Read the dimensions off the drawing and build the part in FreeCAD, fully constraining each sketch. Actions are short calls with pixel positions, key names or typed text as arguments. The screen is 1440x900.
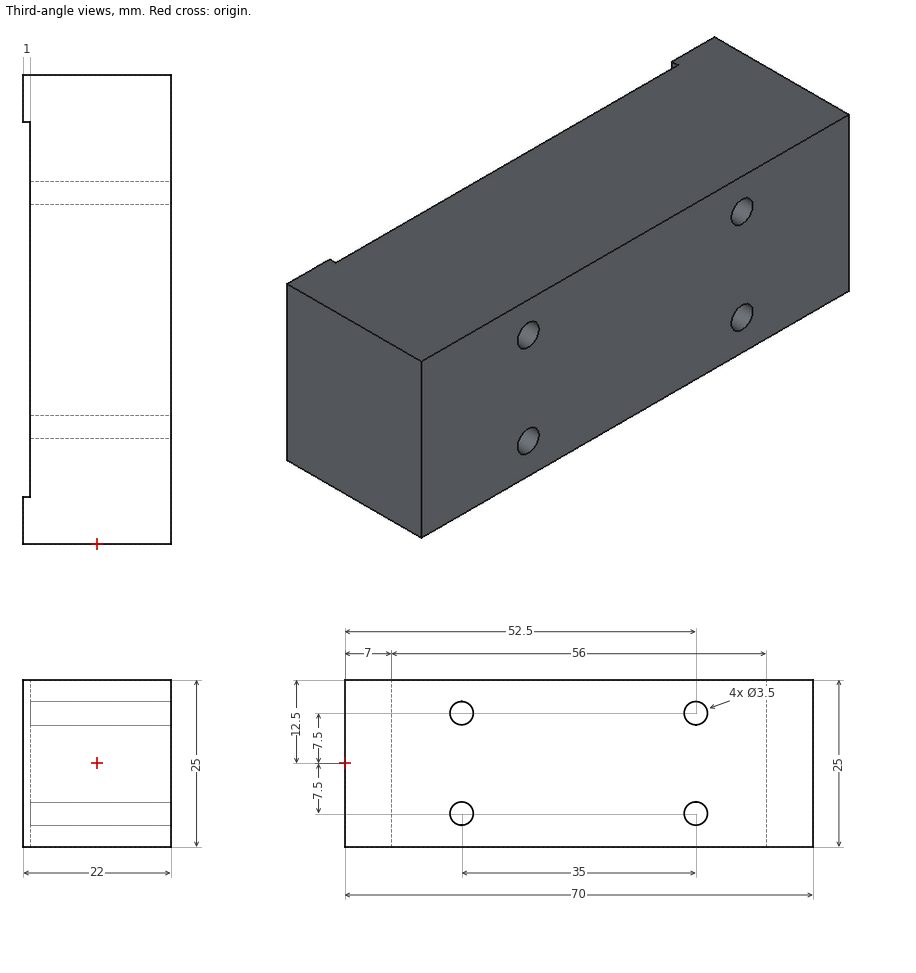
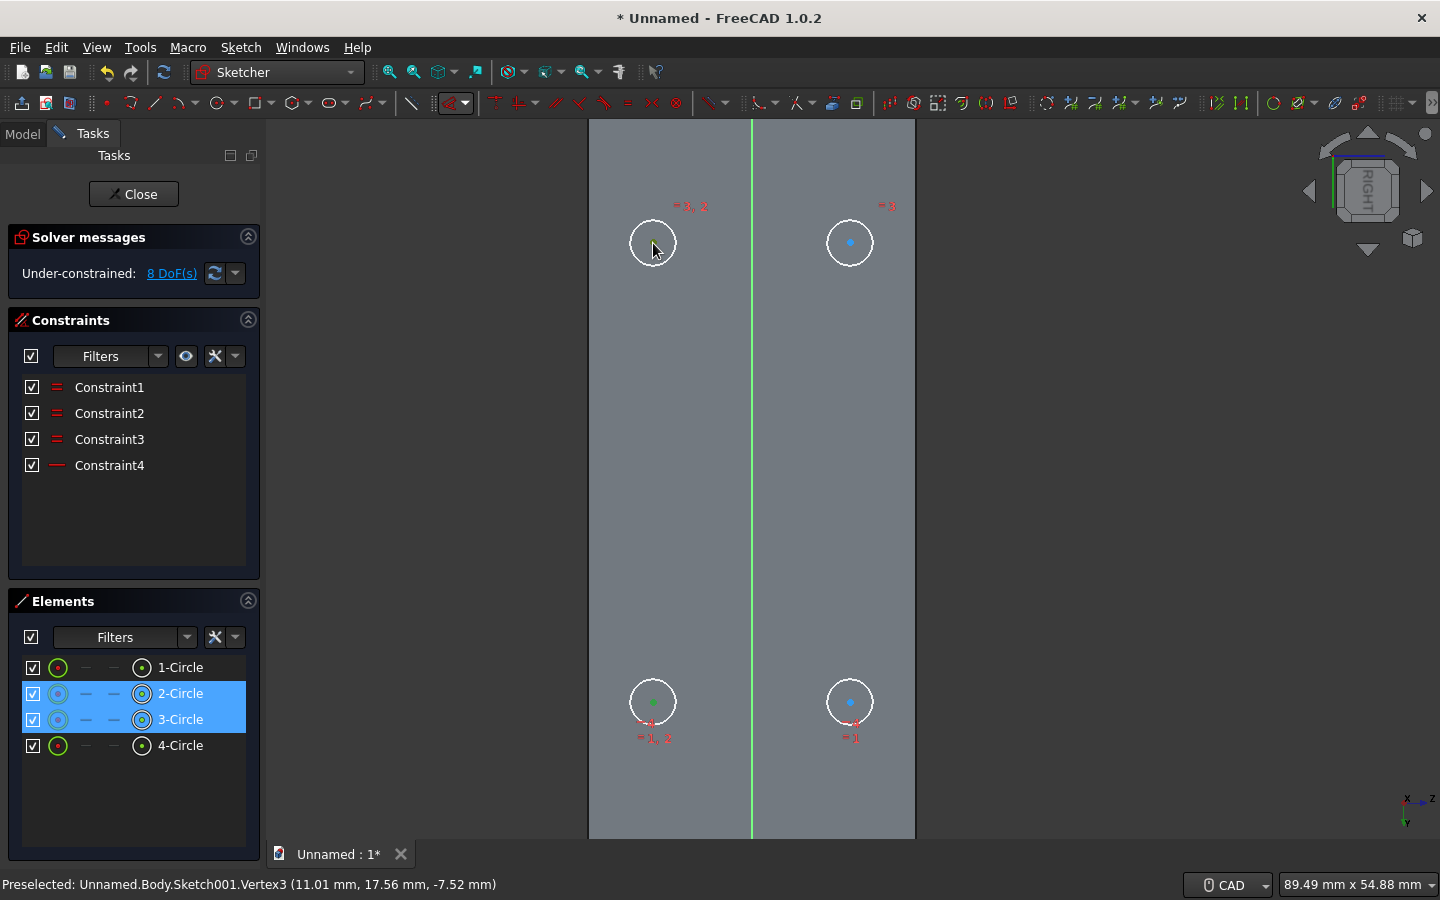
click(538, 104)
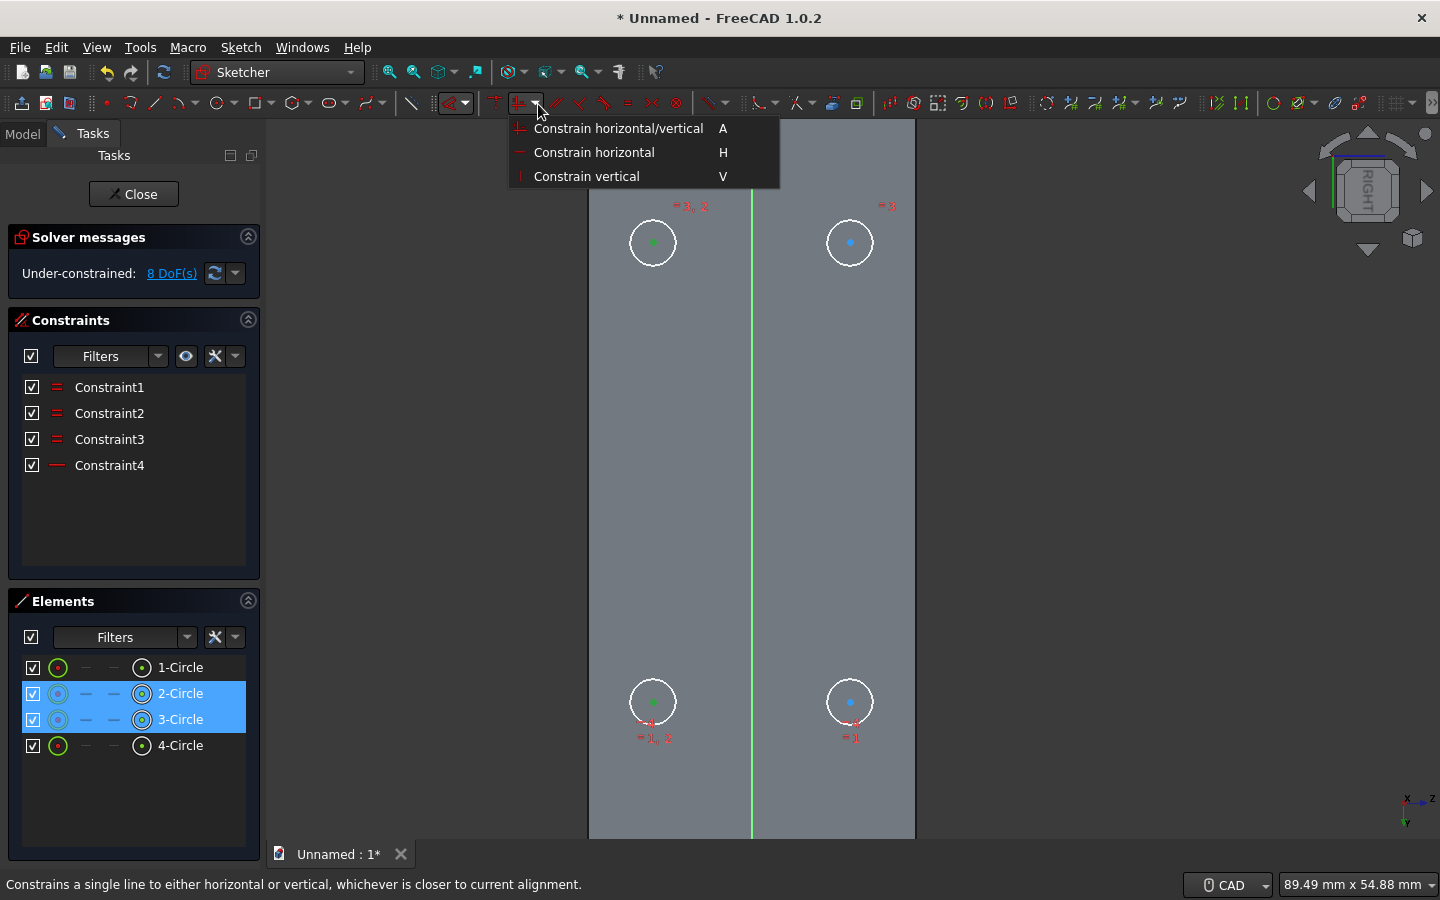
click(644, 176)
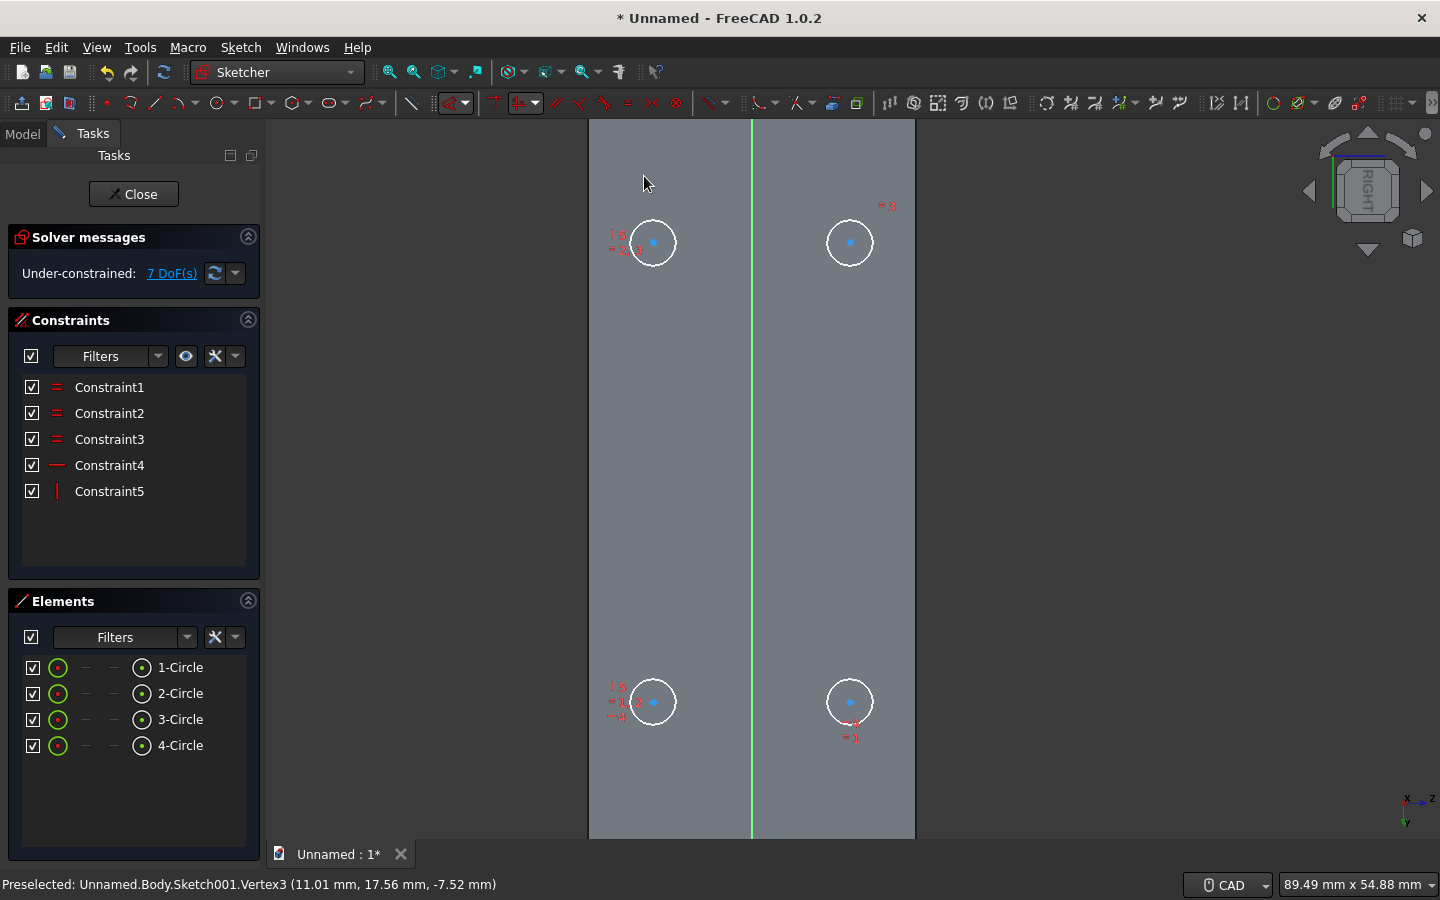
click(850, 702)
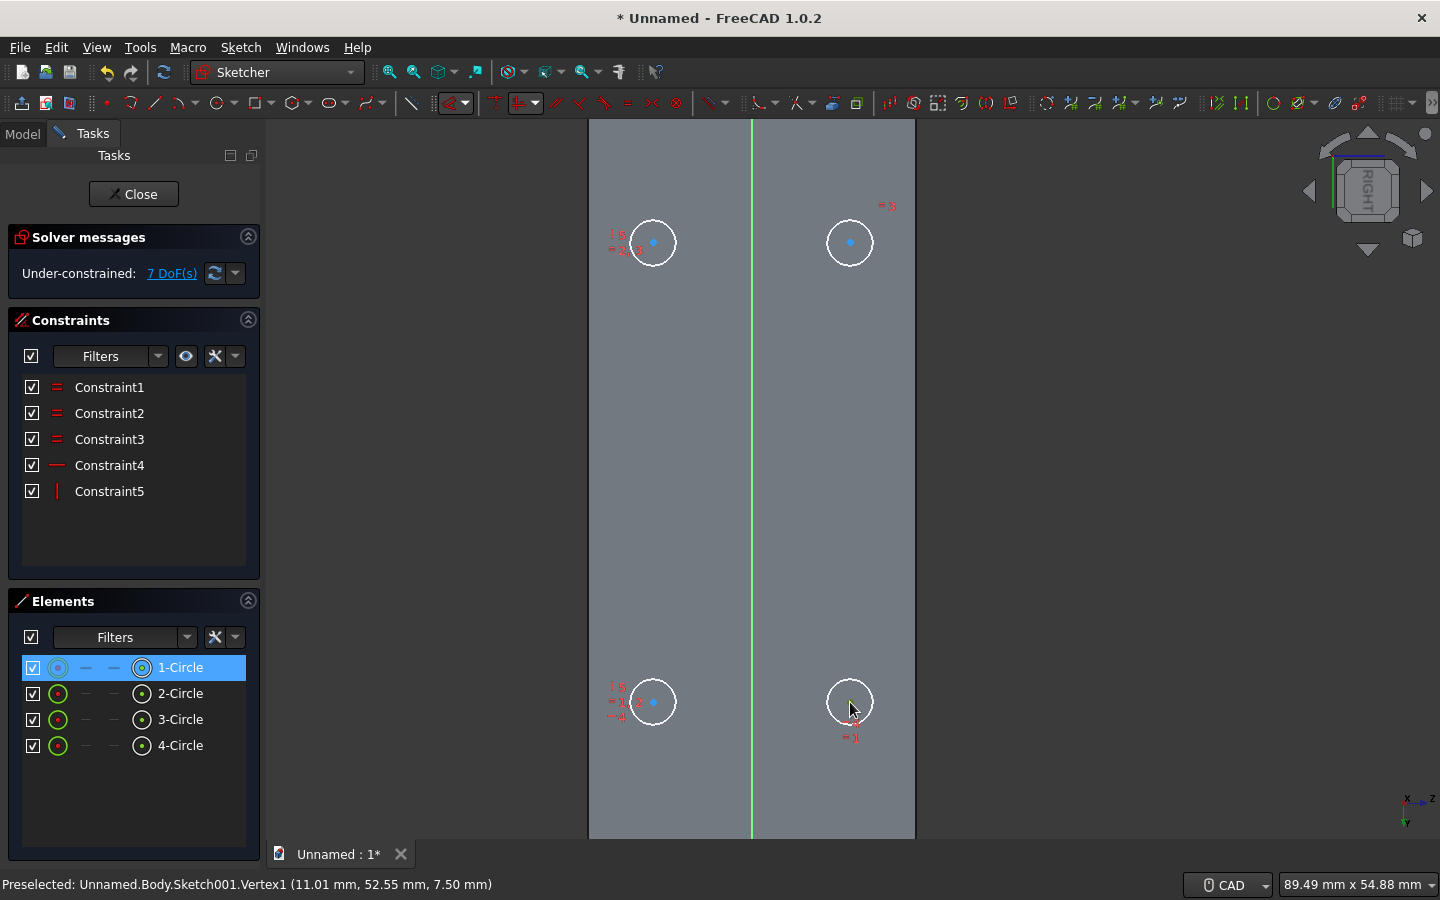
click(850, 243)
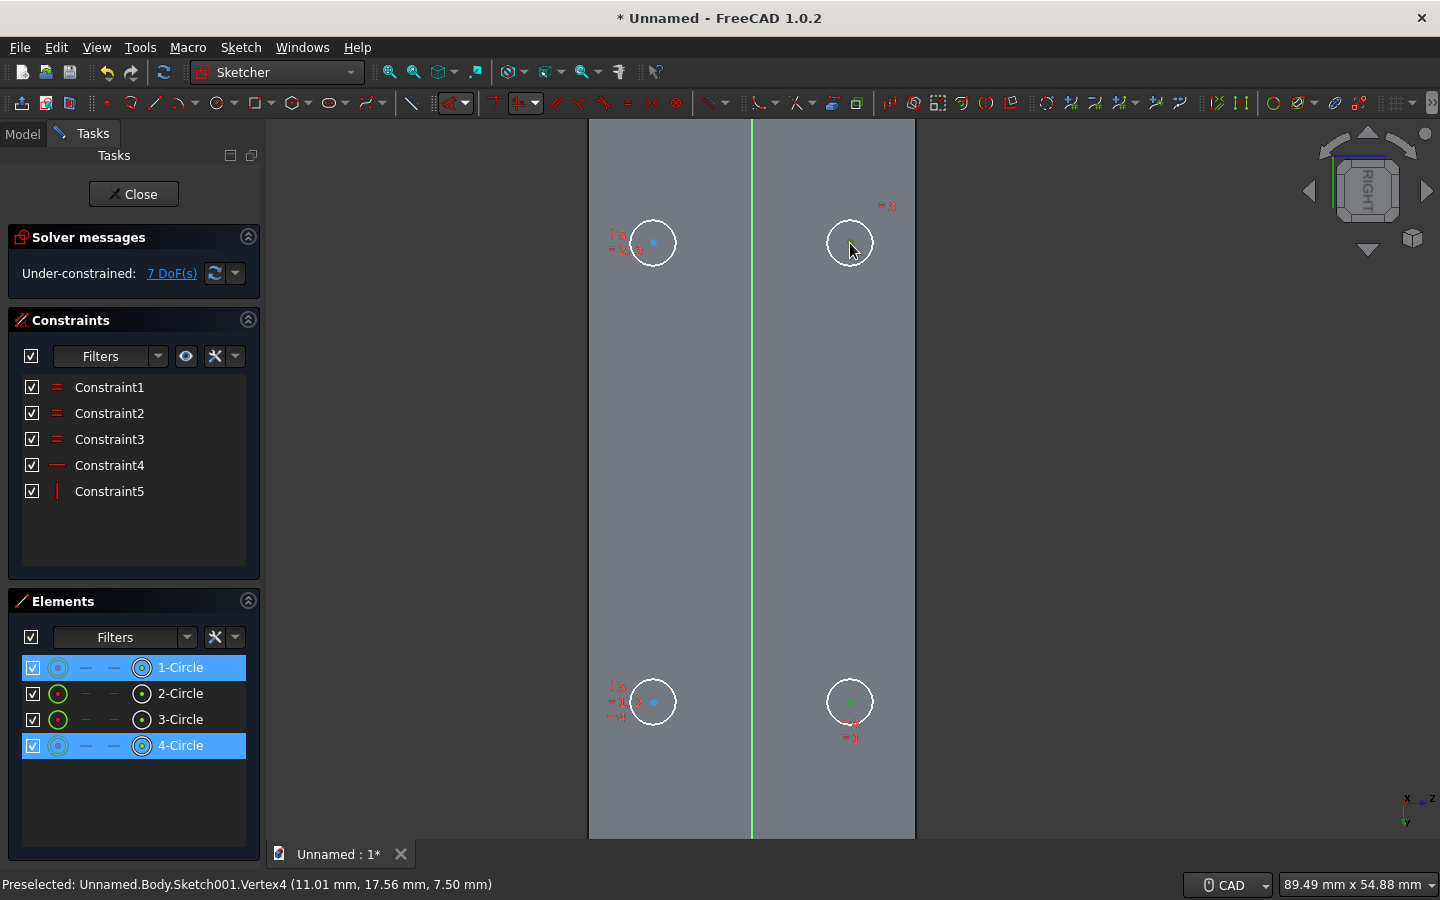
key(v)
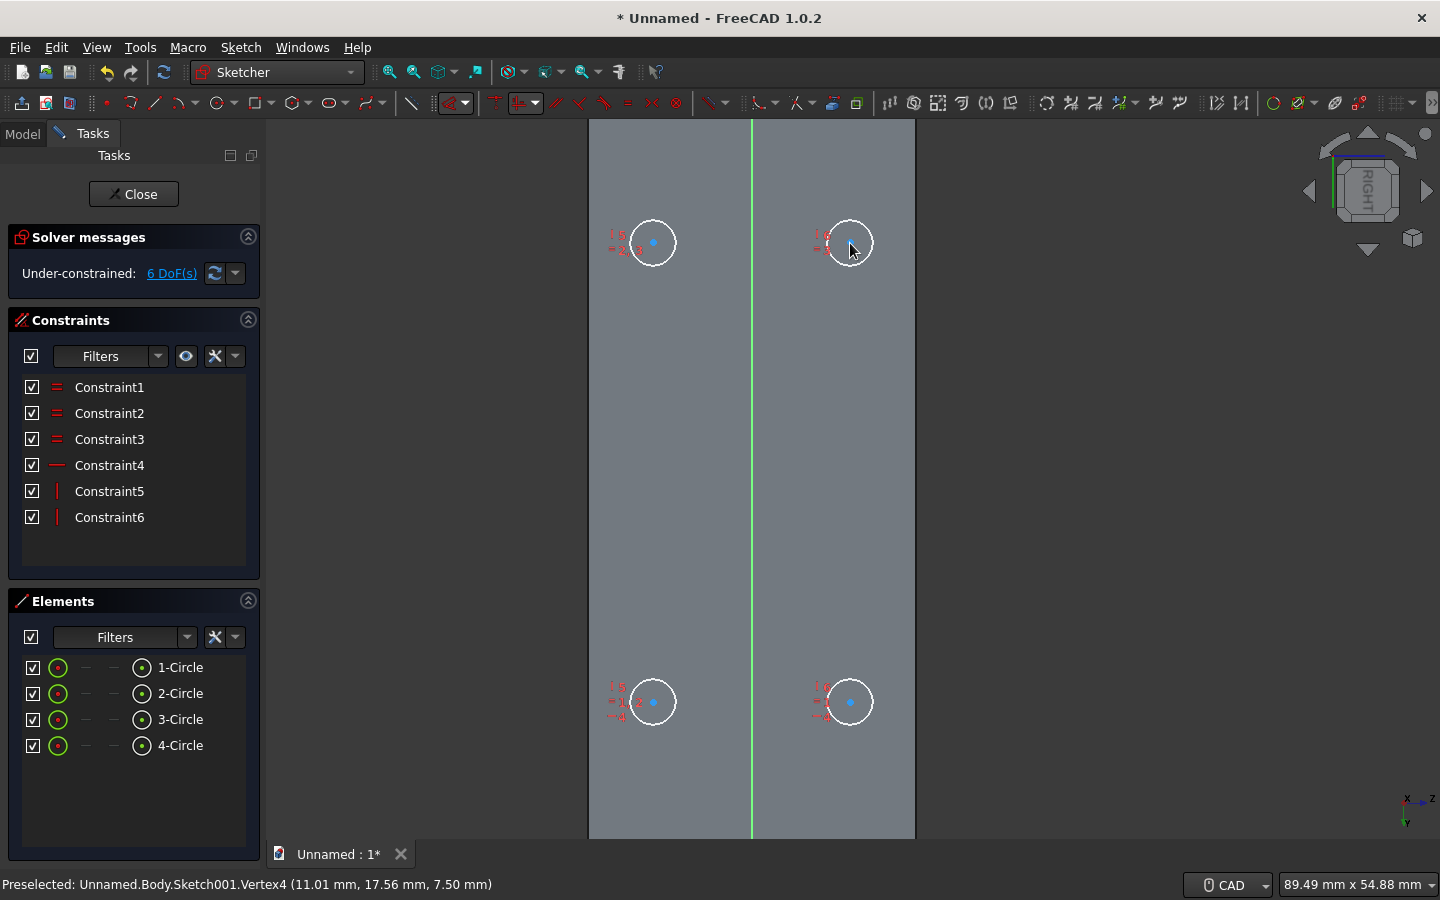
click(653, 243)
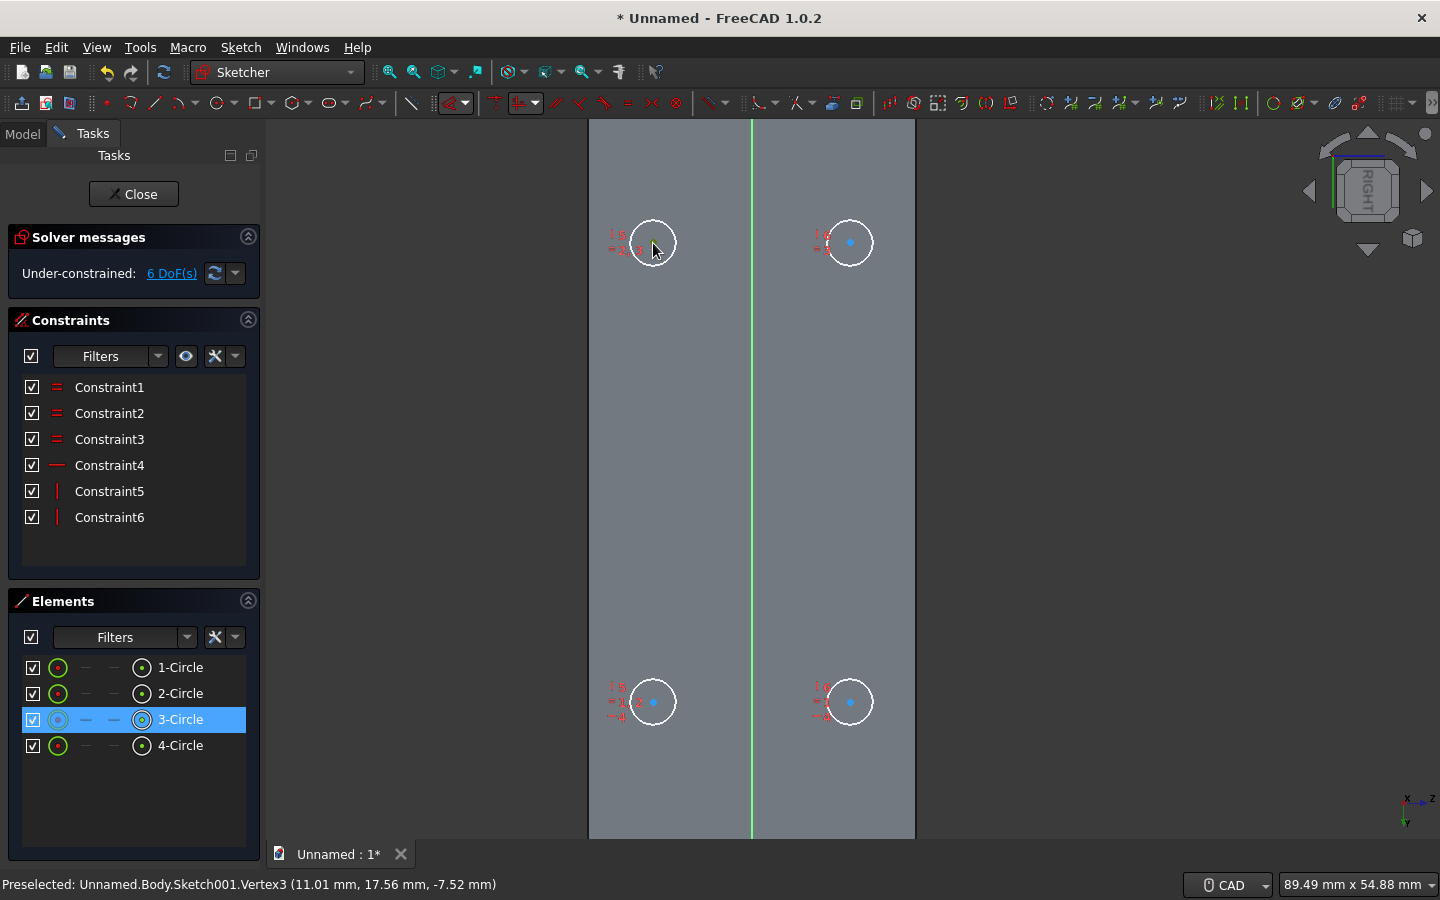
click(850, 243)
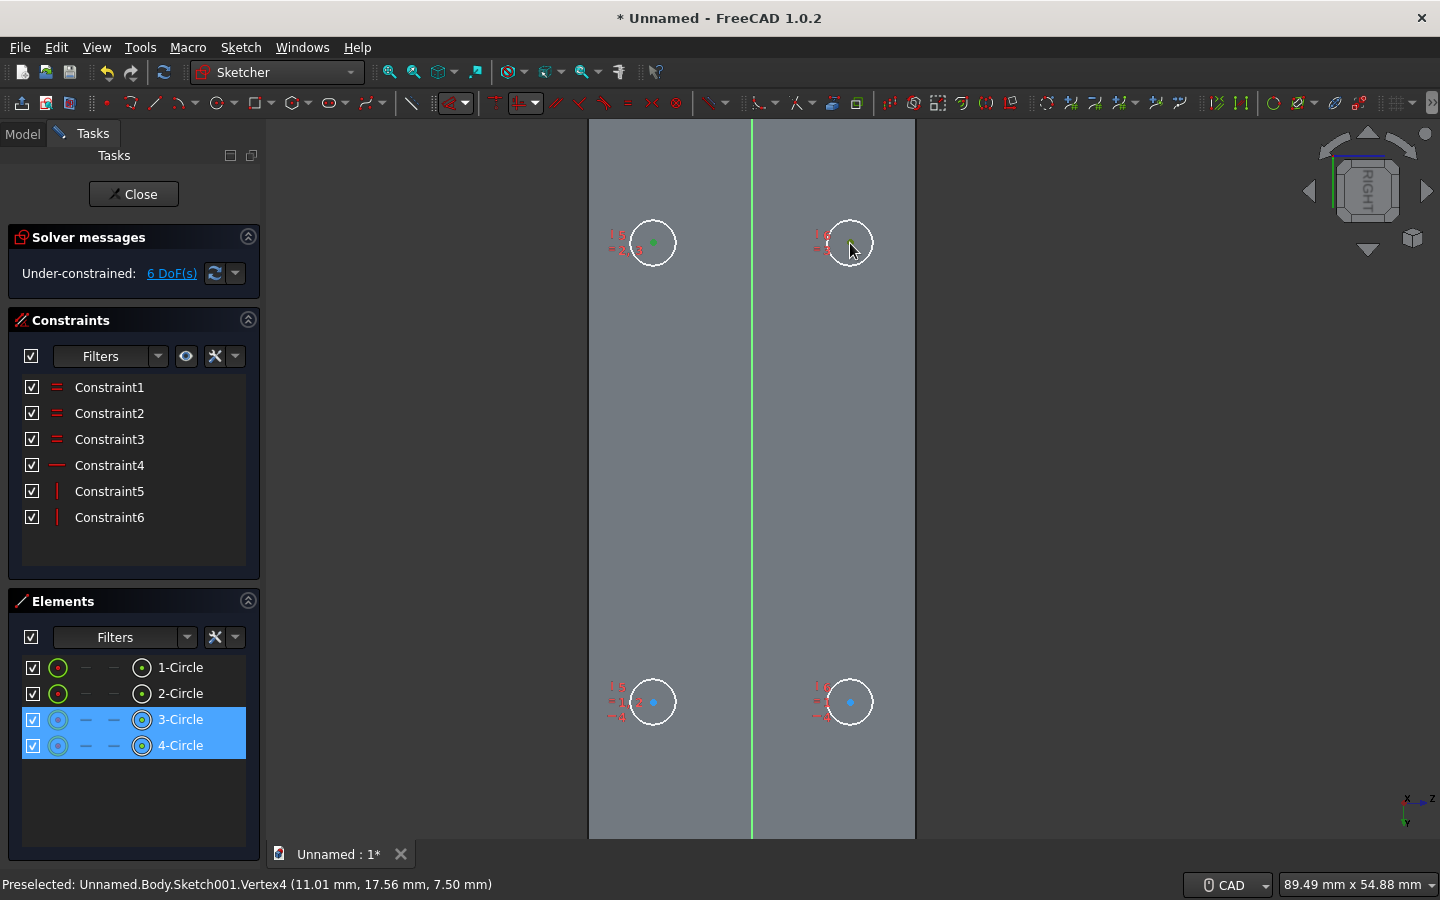
click(538, 104)